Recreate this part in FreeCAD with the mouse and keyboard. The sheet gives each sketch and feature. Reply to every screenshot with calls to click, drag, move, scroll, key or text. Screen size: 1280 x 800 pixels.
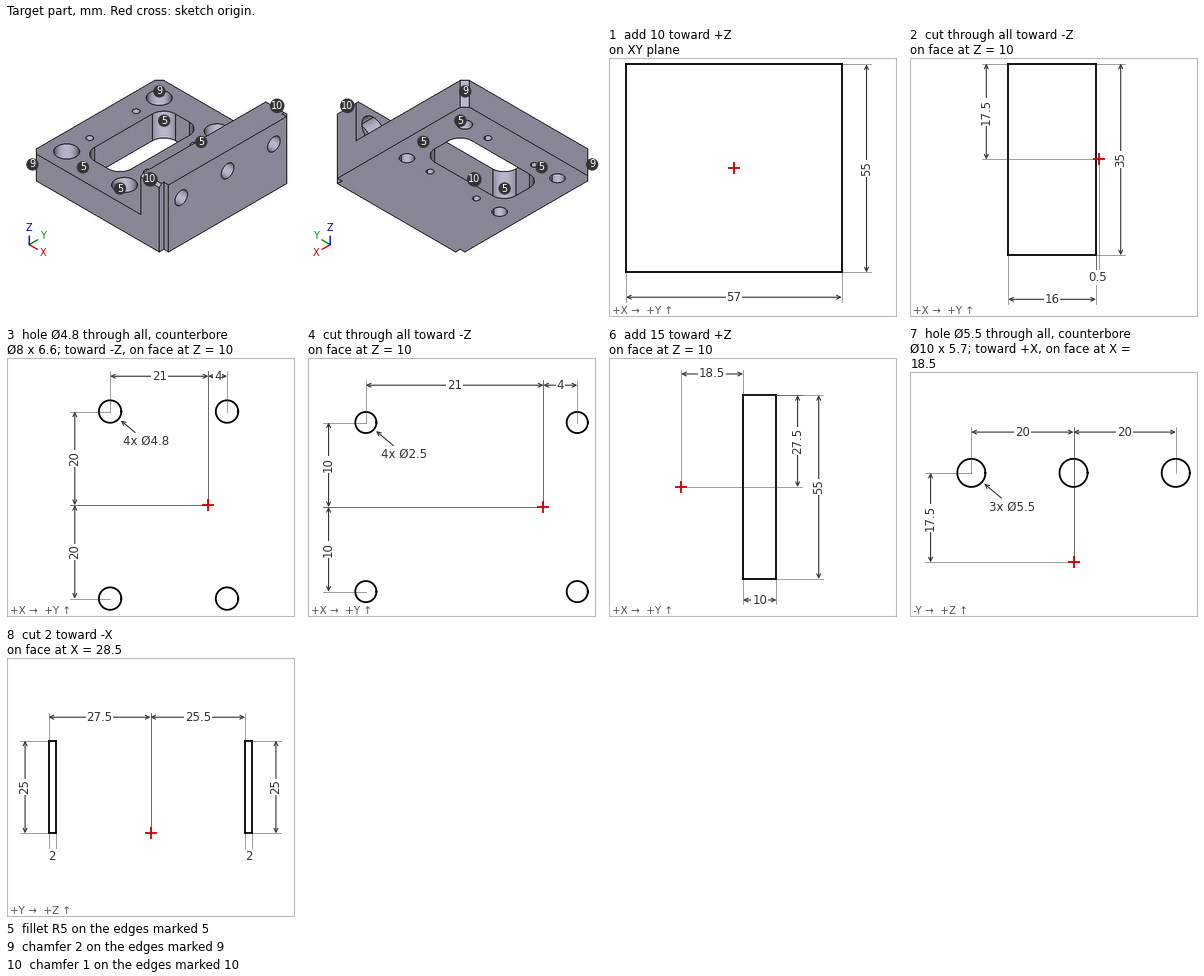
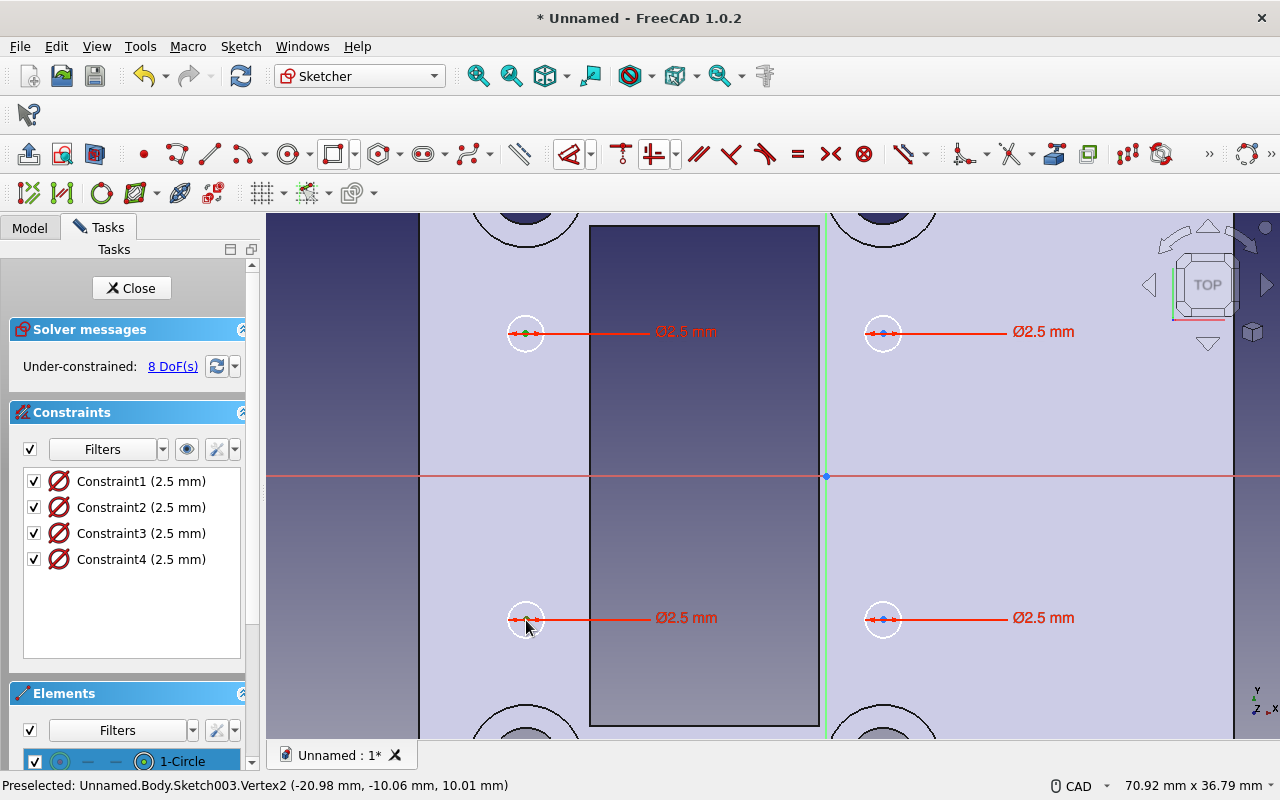
key(v)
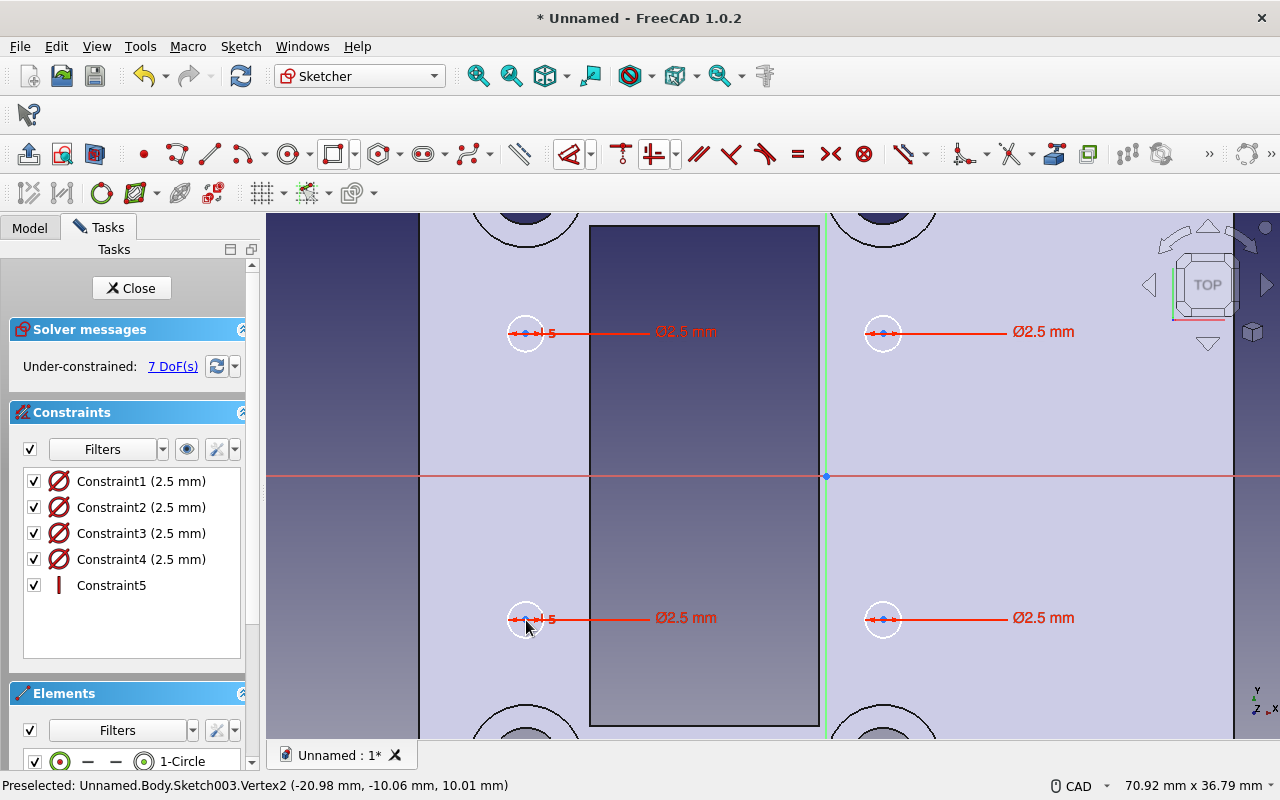
click(526, 334)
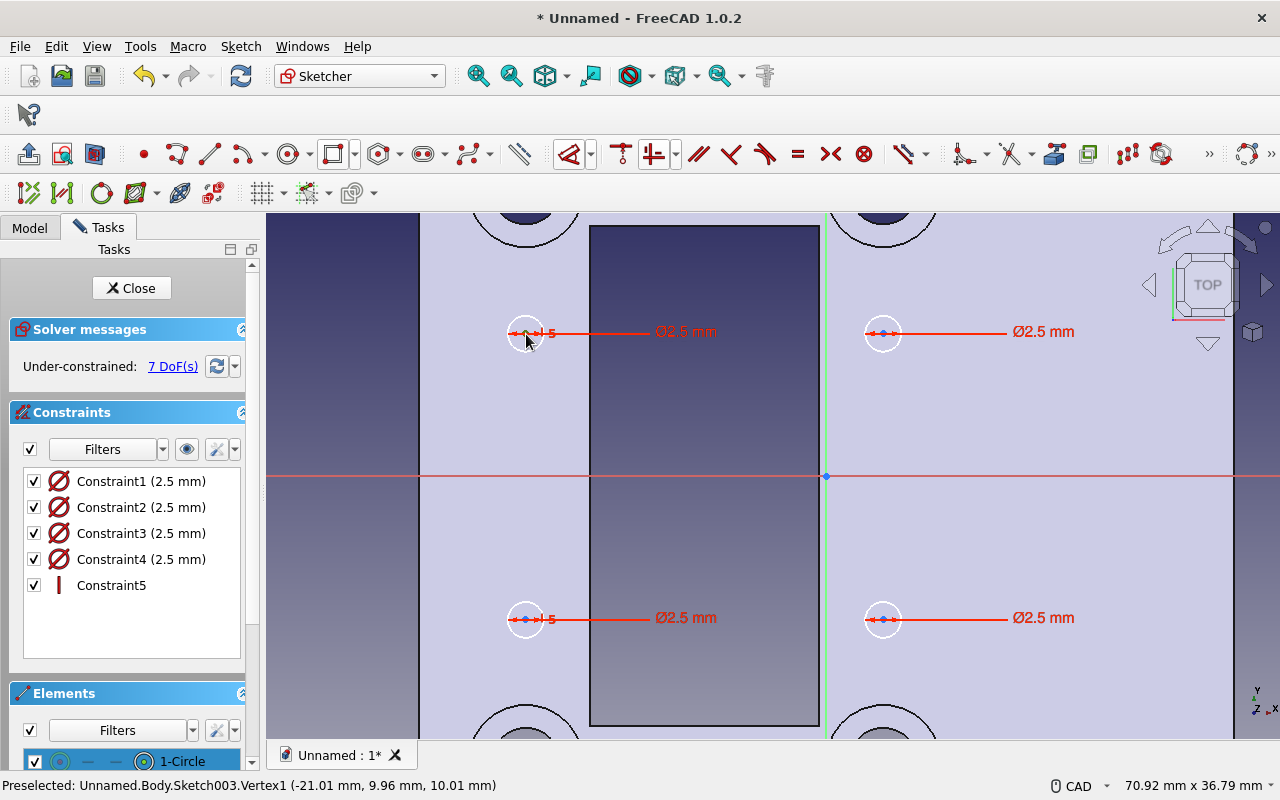
click(883, 334)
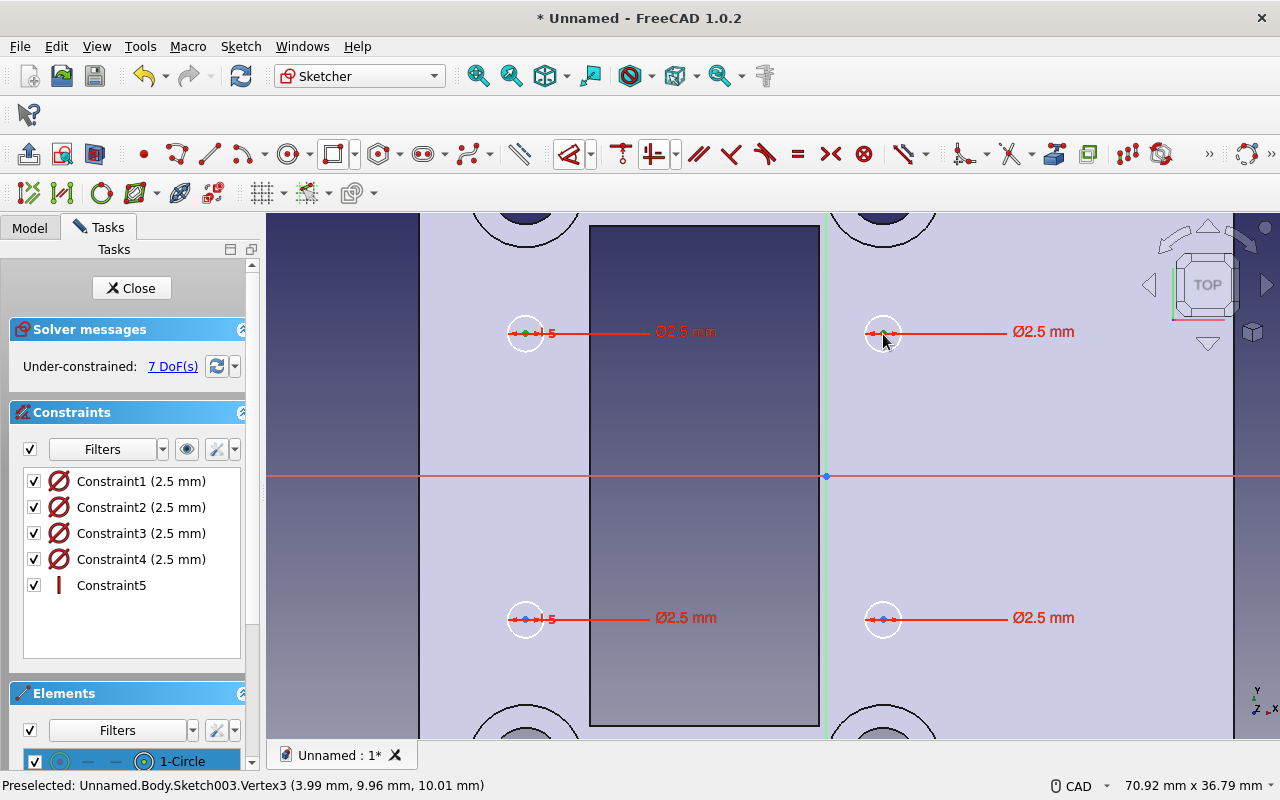
key(h)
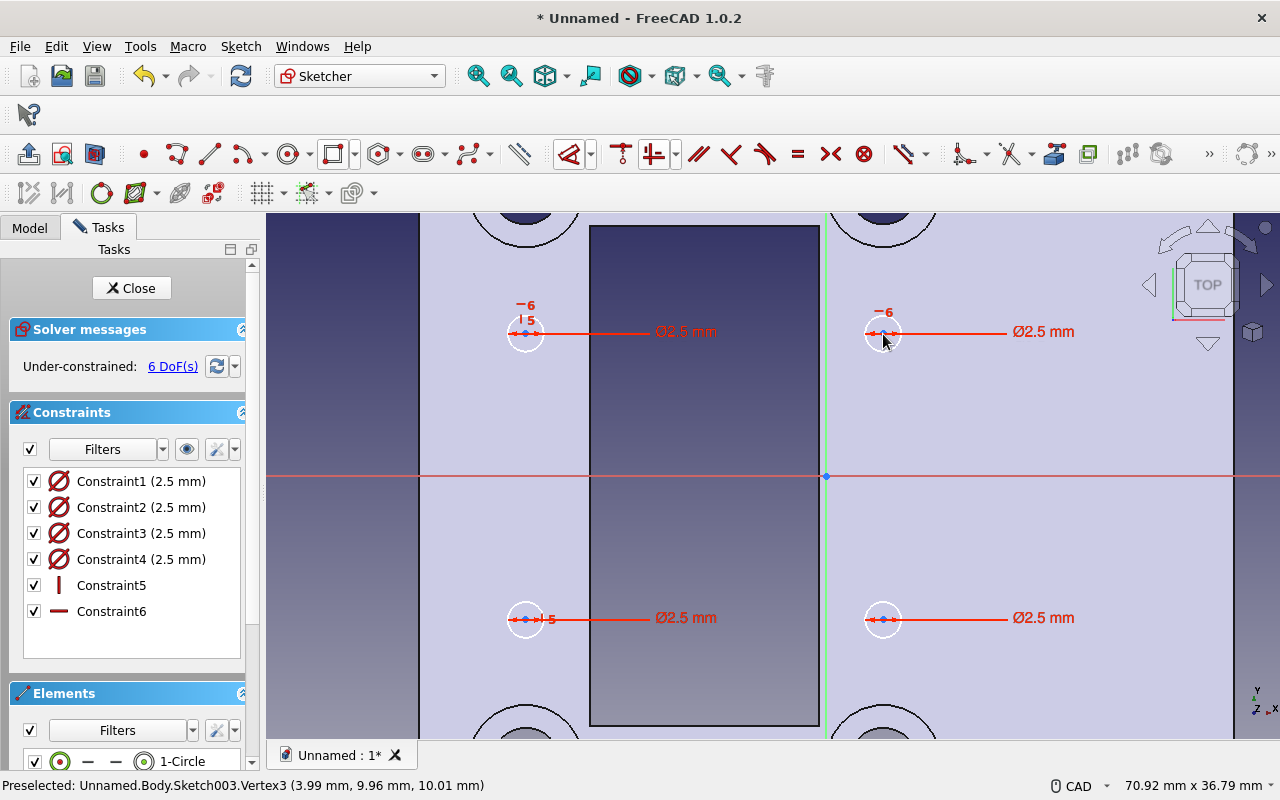
click(883, 334)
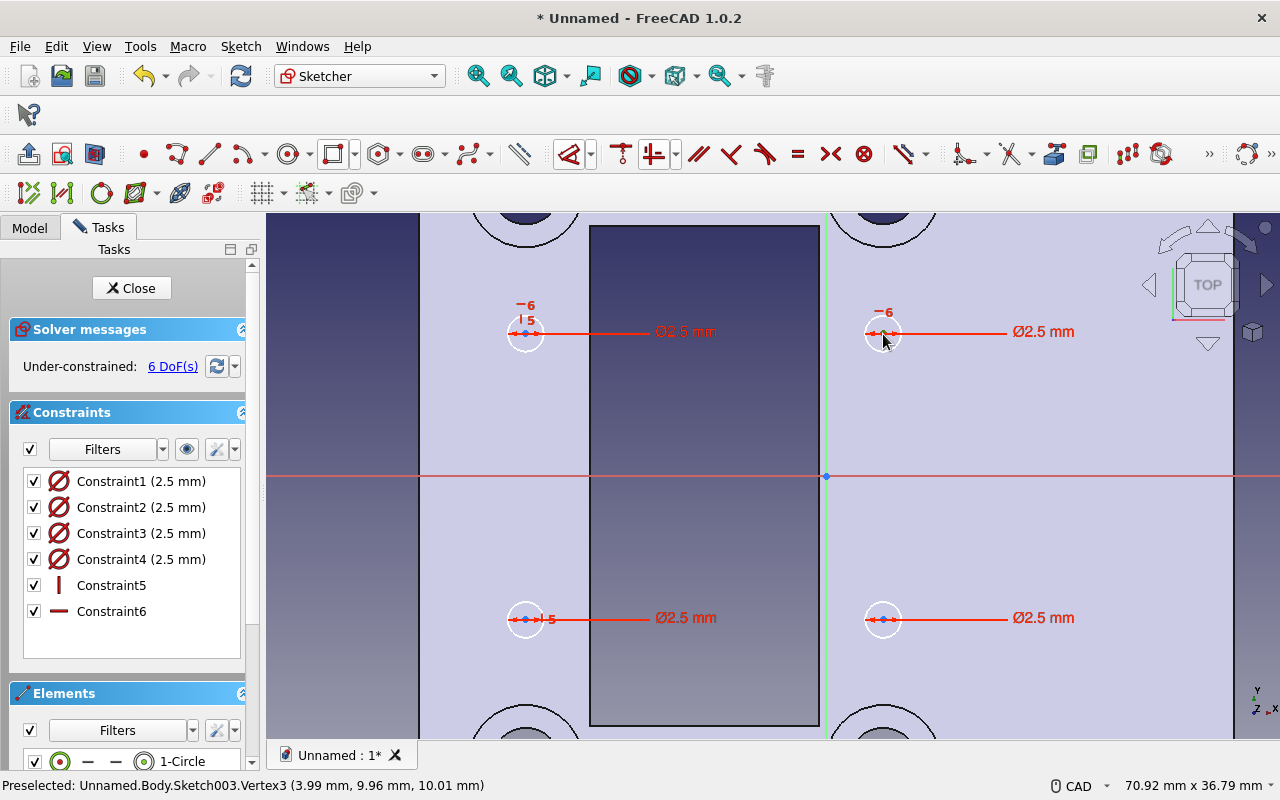
click(883, 620)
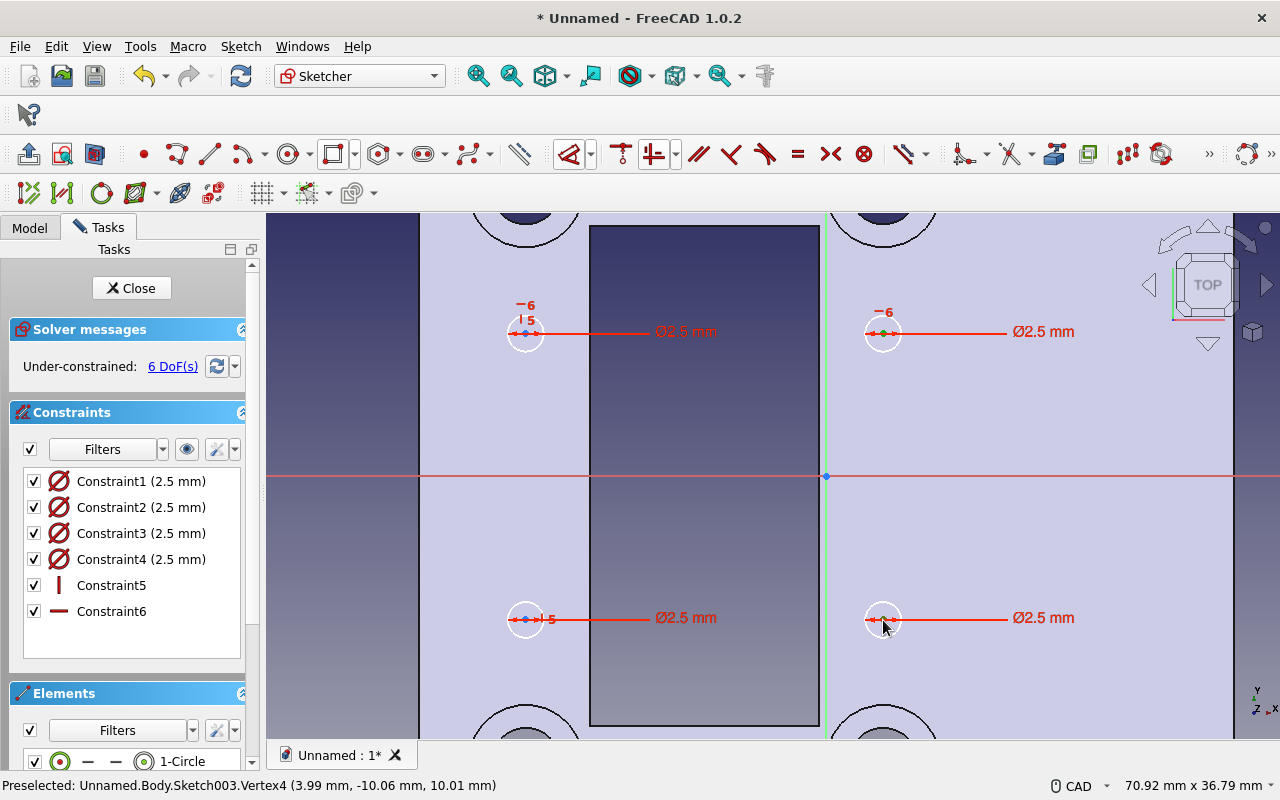
click(676, 154)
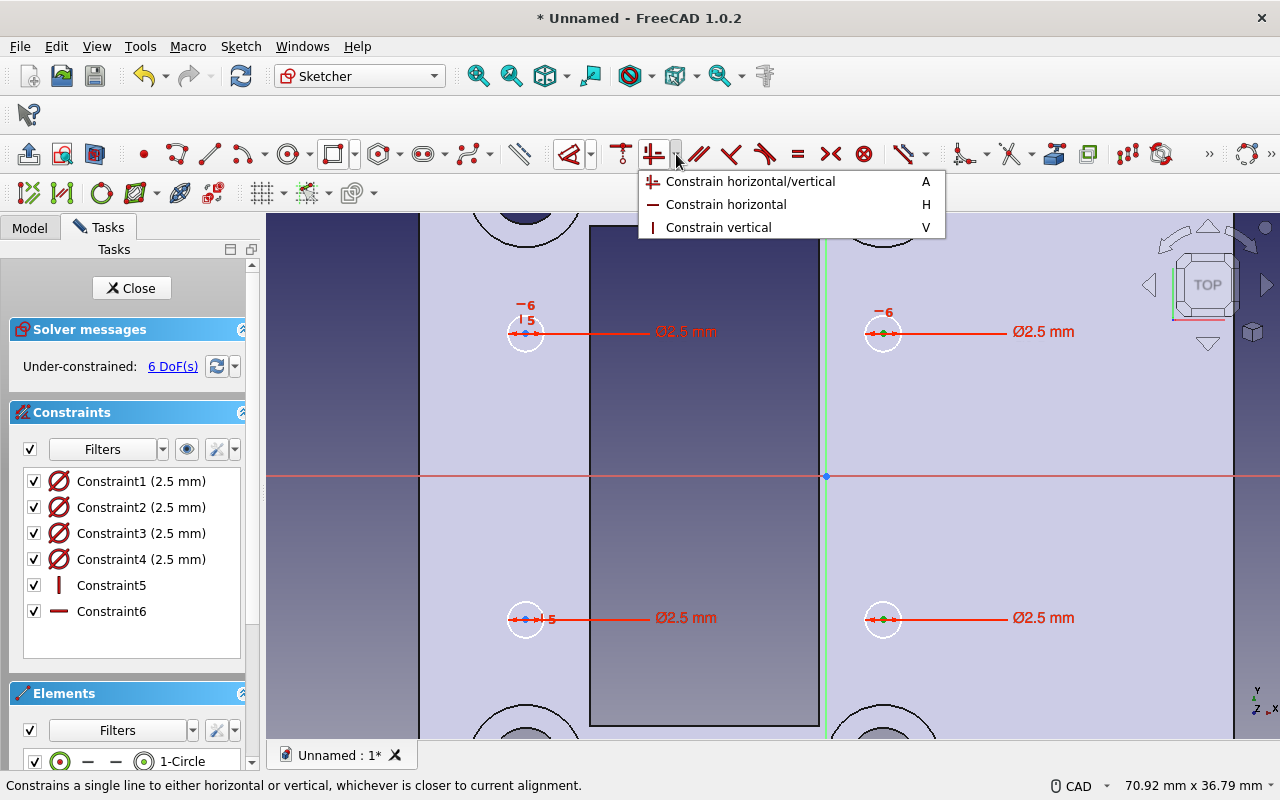
click(792, 228)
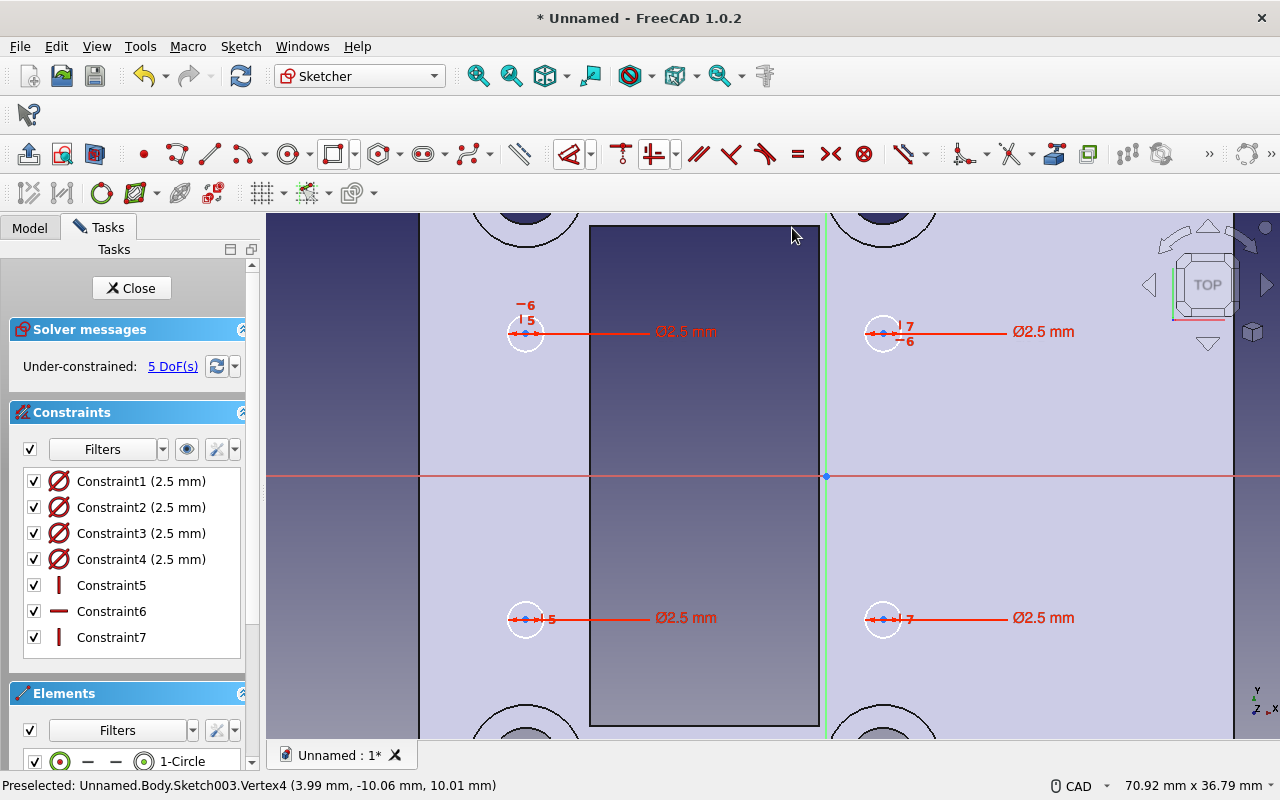
click(526, 620)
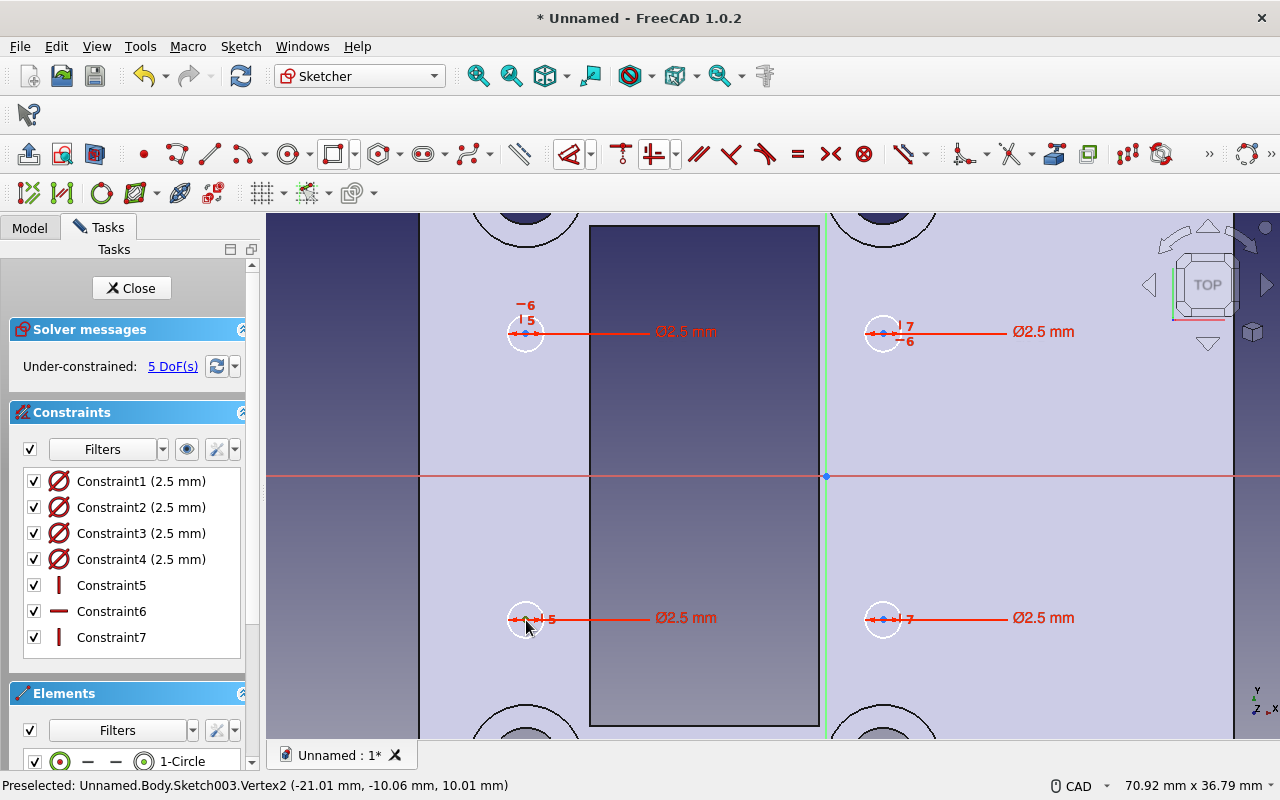
click(883, 620)